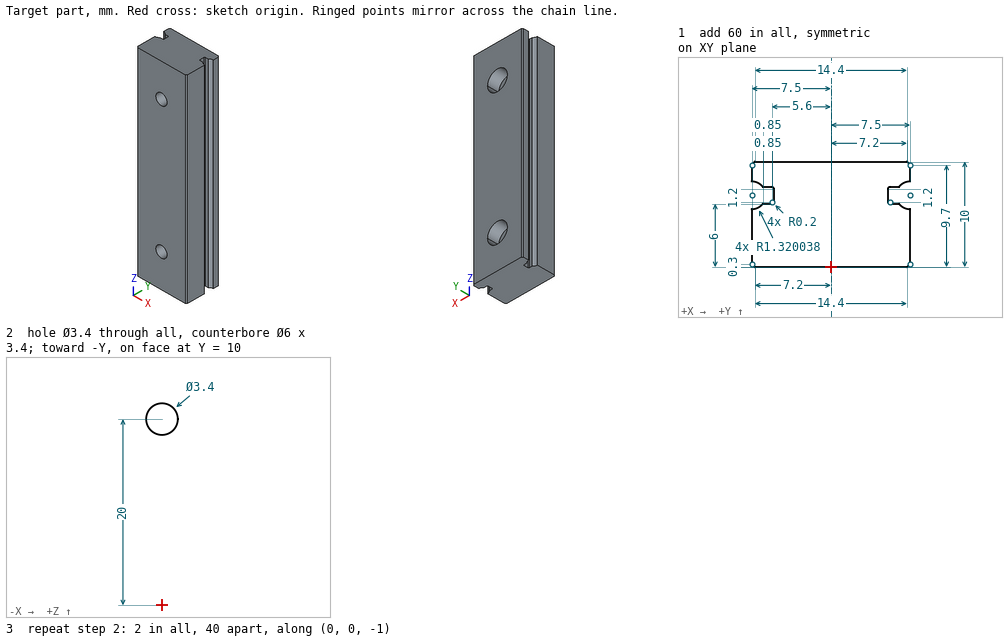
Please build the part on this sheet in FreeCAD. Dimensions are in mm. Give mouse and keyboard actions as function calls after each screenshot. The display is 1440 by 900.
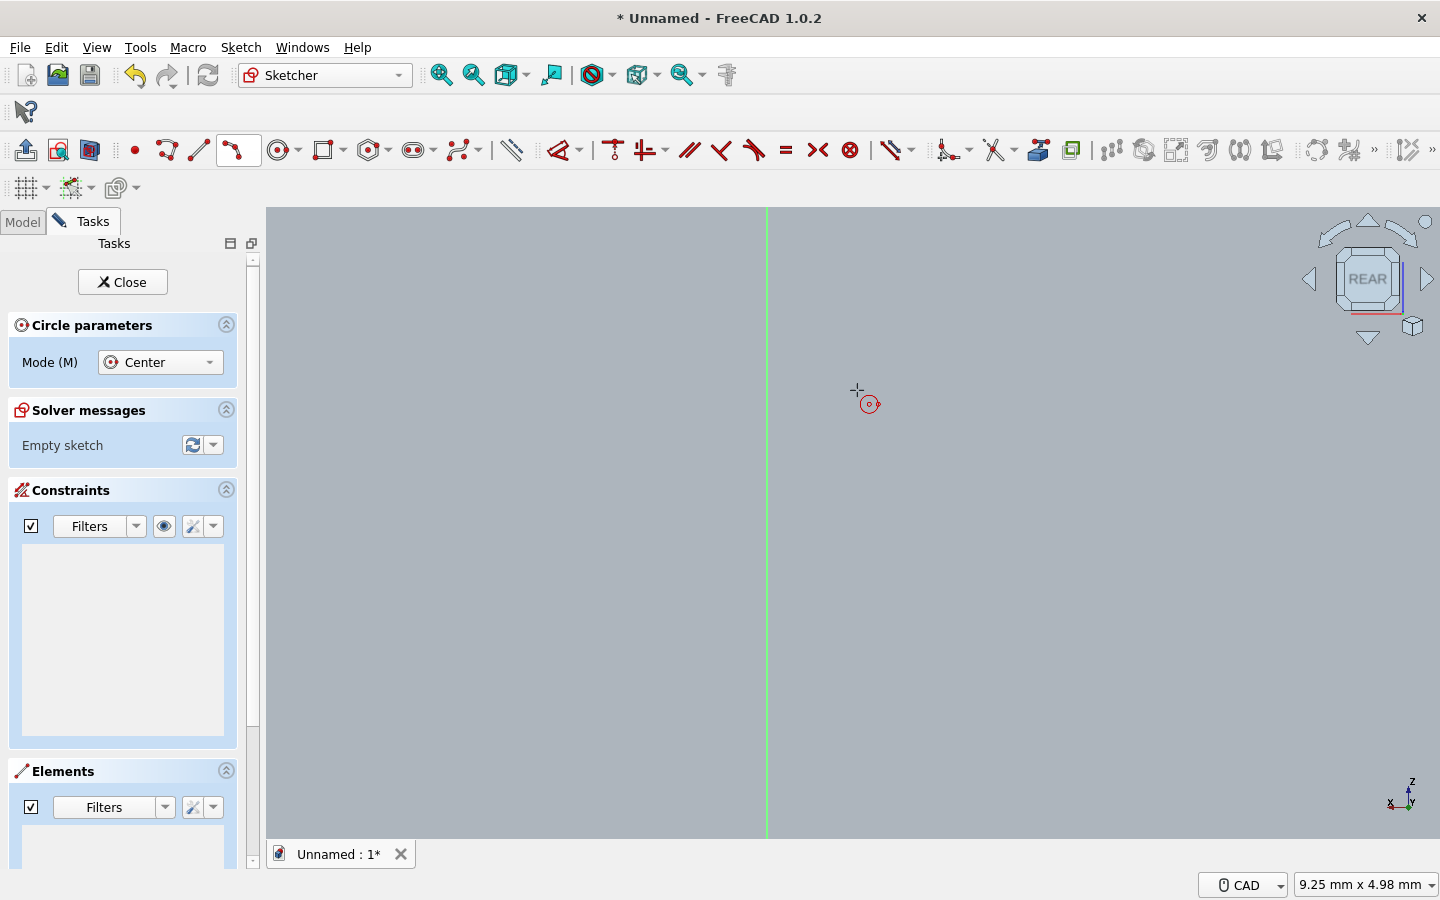
click(767, 517)
move(920, 364)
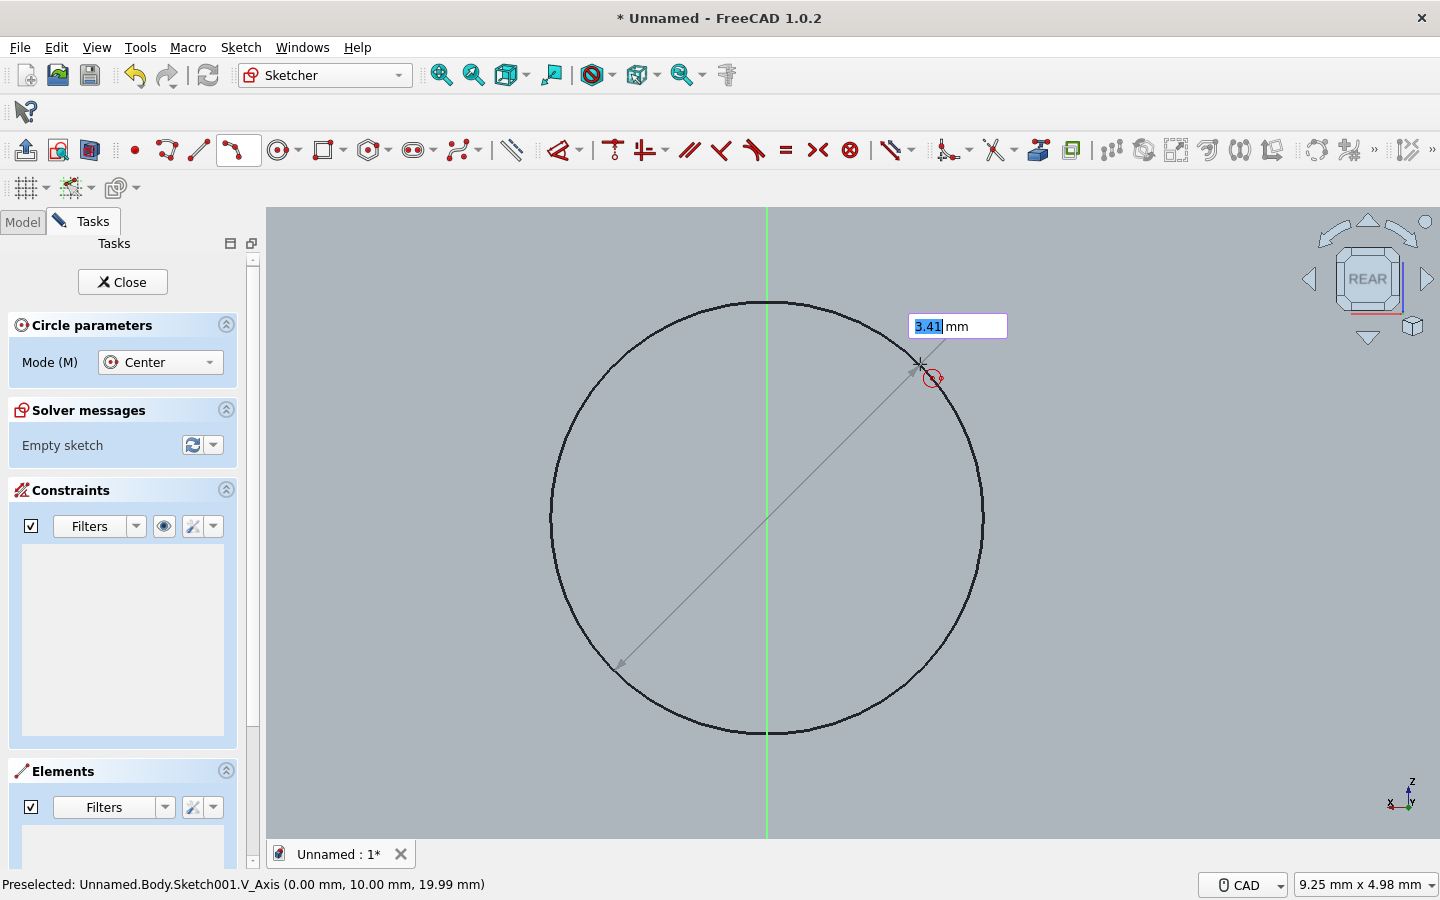
text(3.4)
key(Return)
key(Escape)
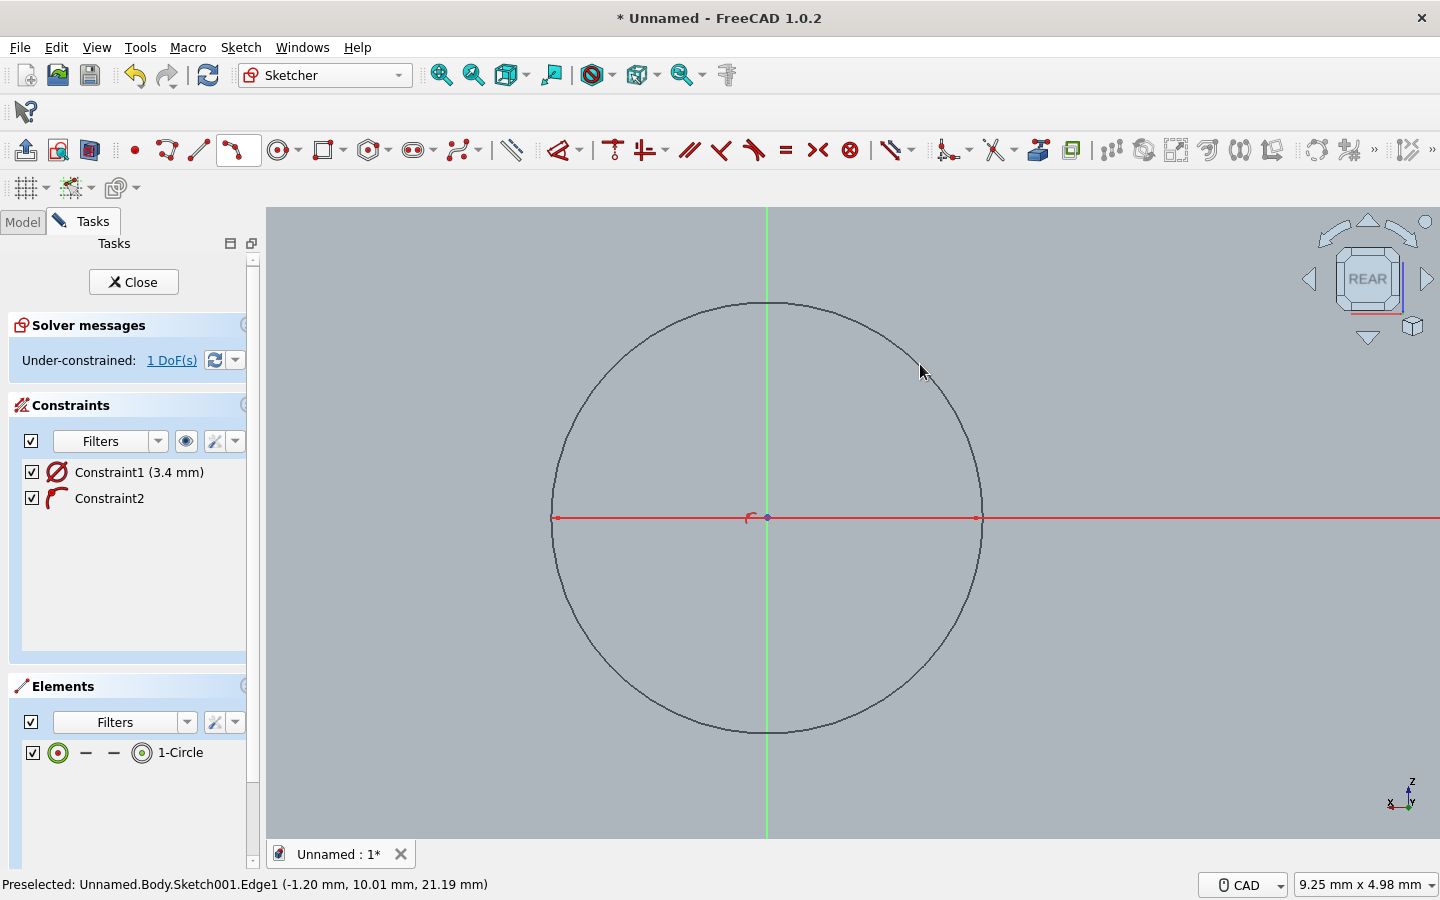
click(558, 150)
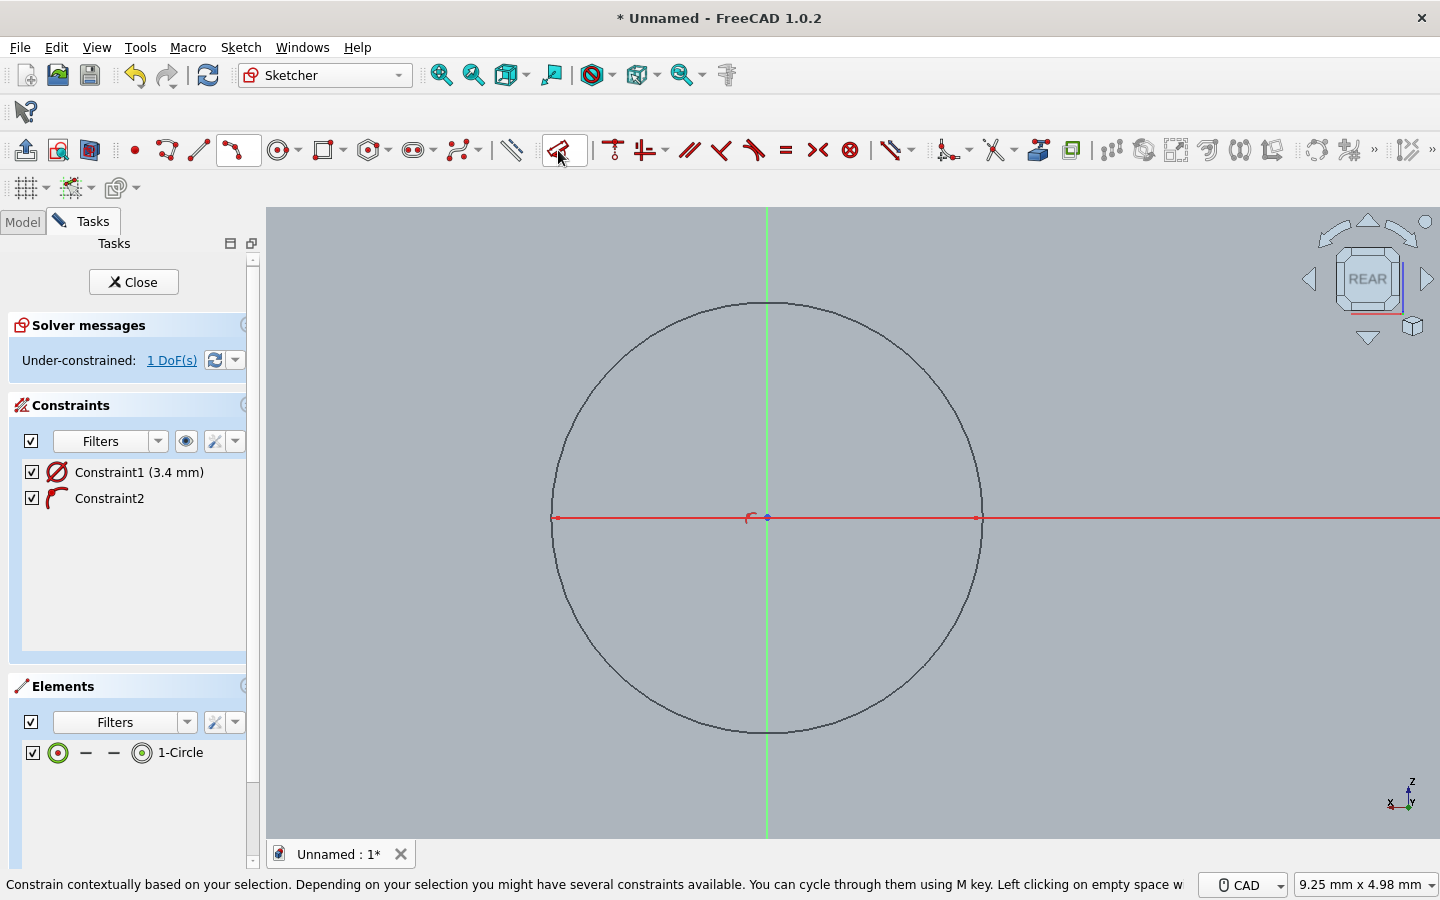
click(767, 518)
click(801, 664)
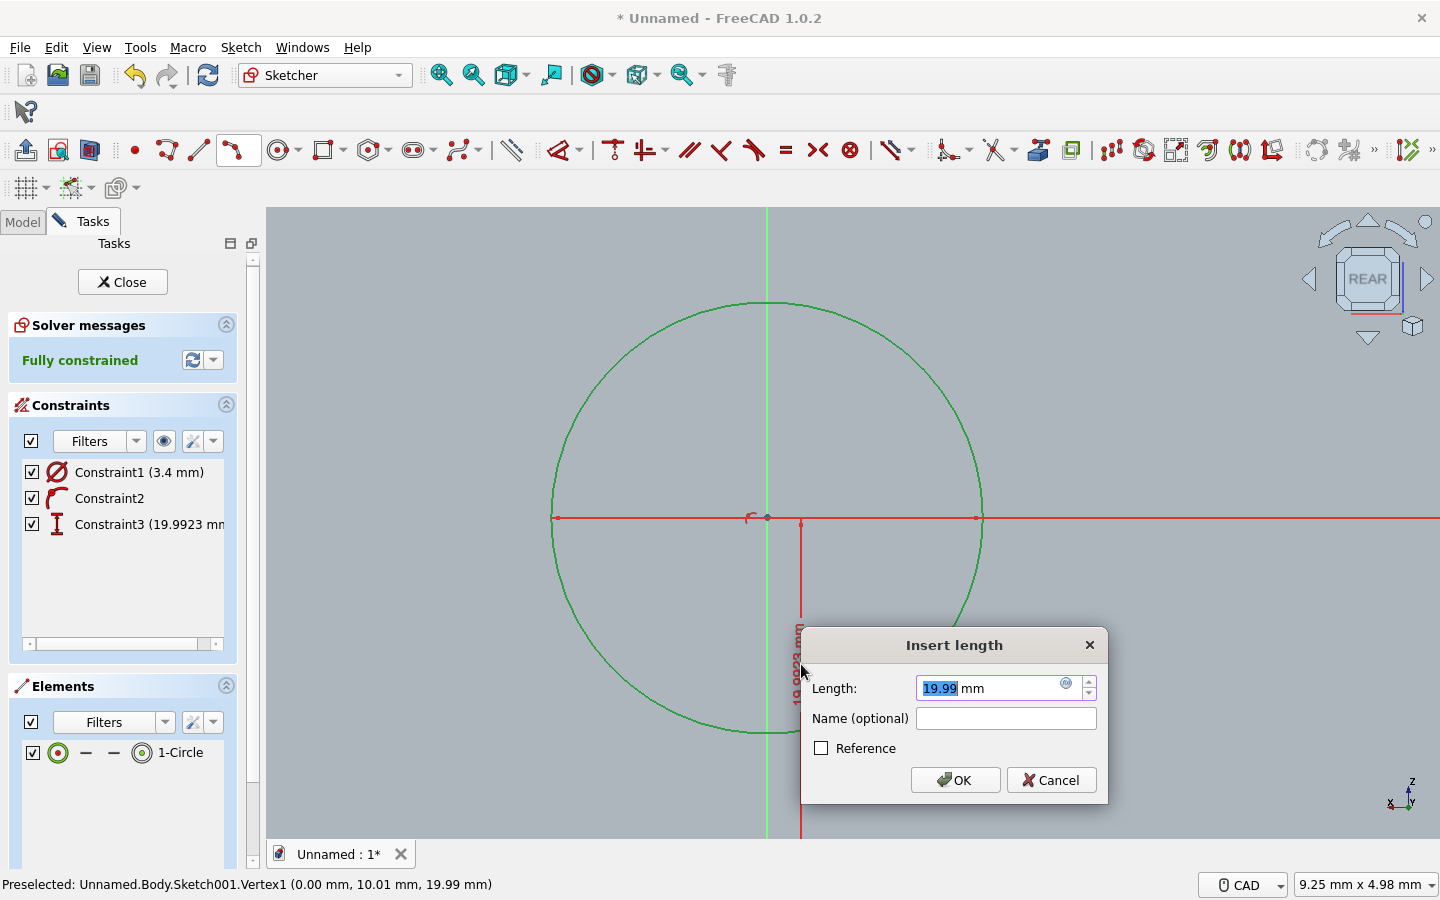
text(20)
key(Return)
key(Escape)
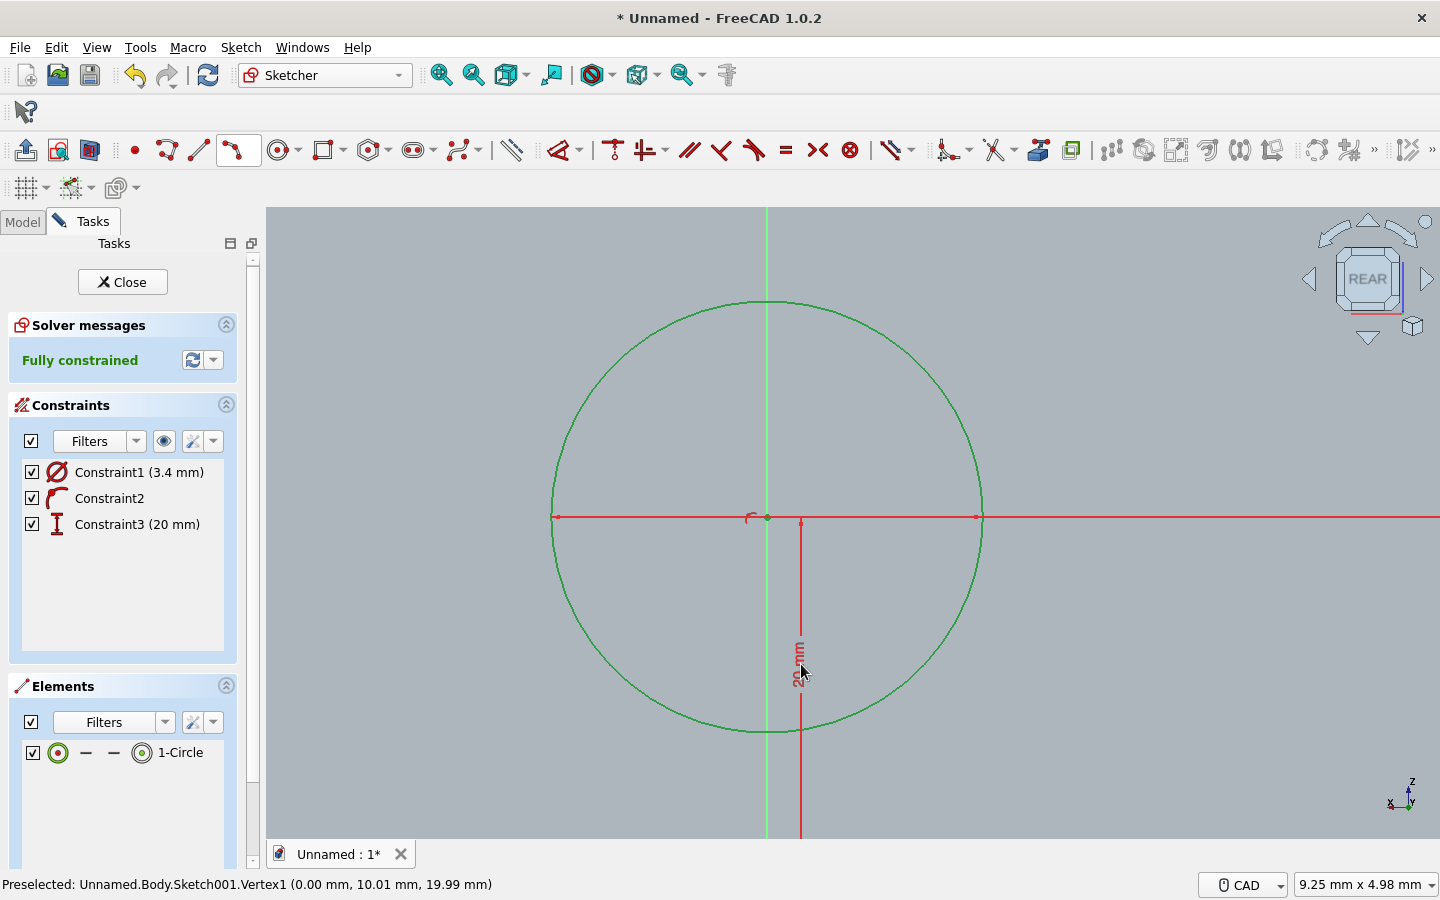
click(123, 282)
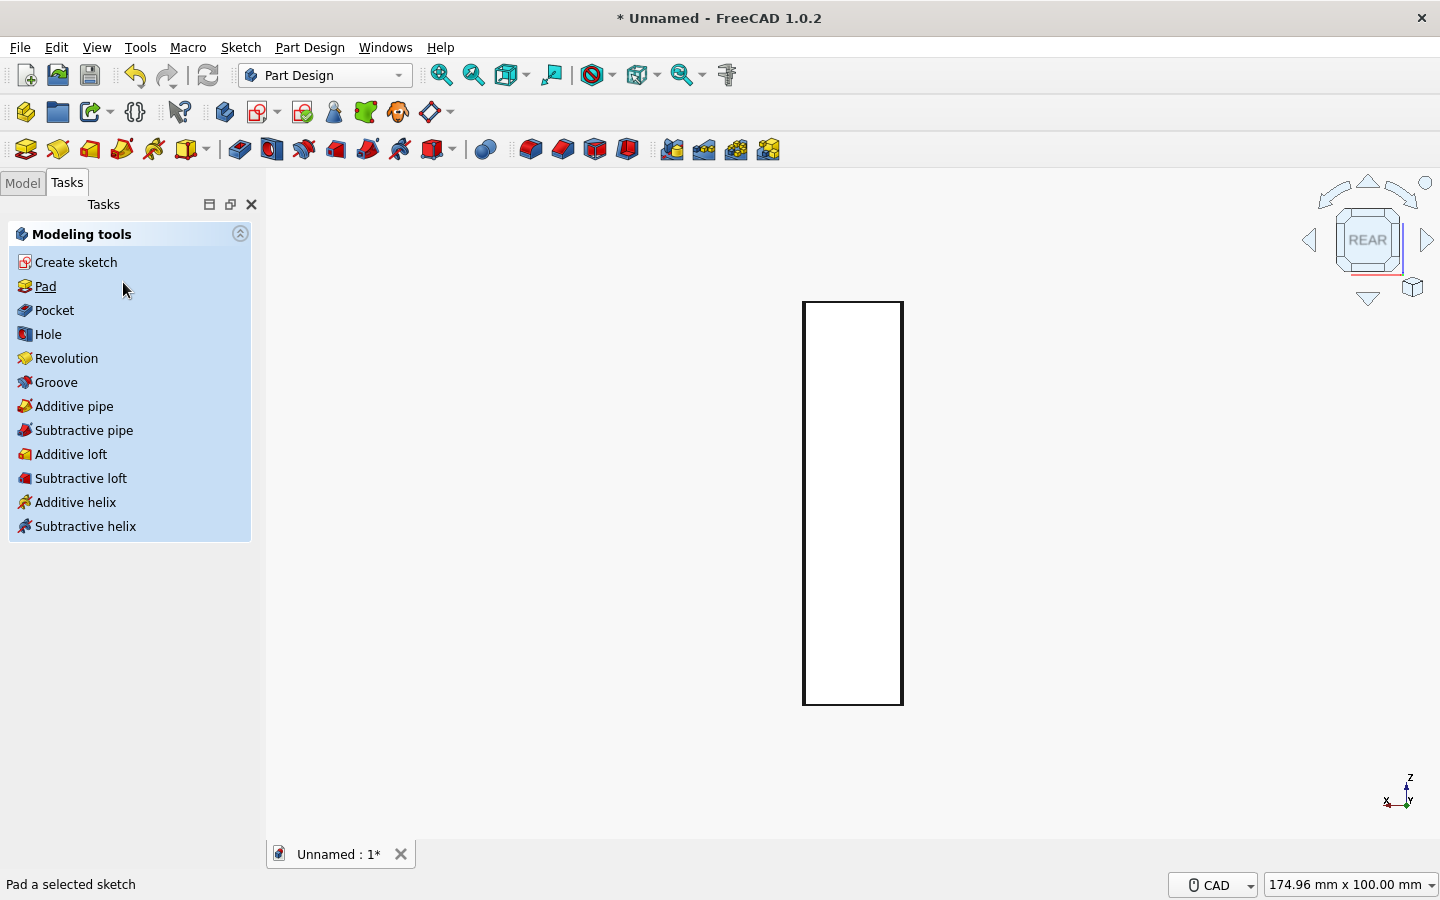
click(272, 150)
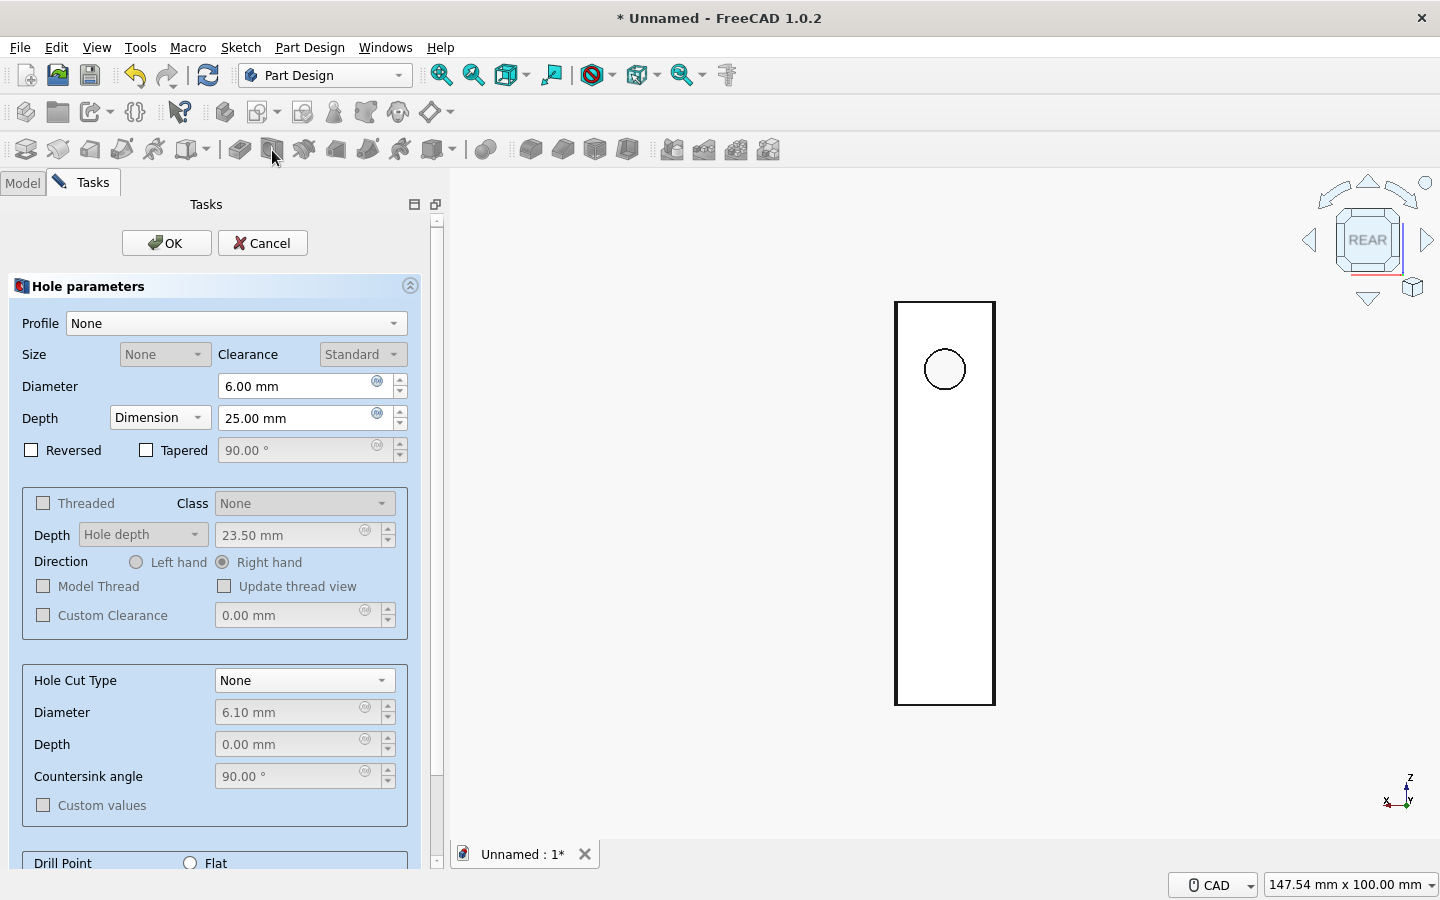
triple_click(305, 386)